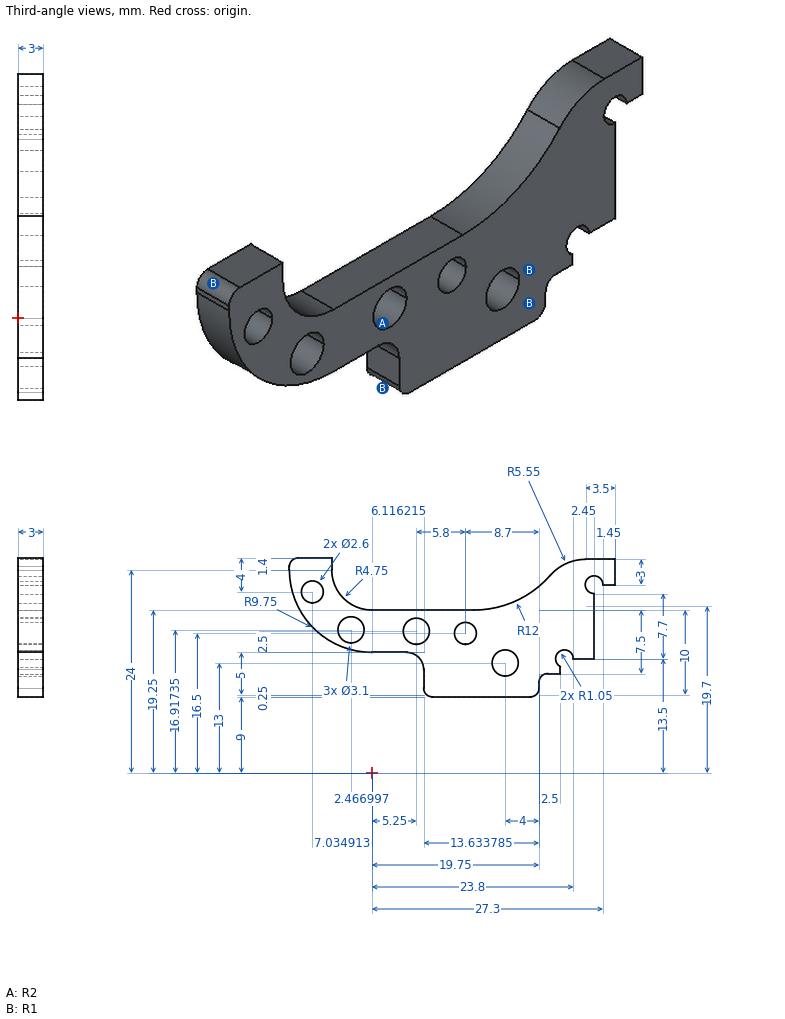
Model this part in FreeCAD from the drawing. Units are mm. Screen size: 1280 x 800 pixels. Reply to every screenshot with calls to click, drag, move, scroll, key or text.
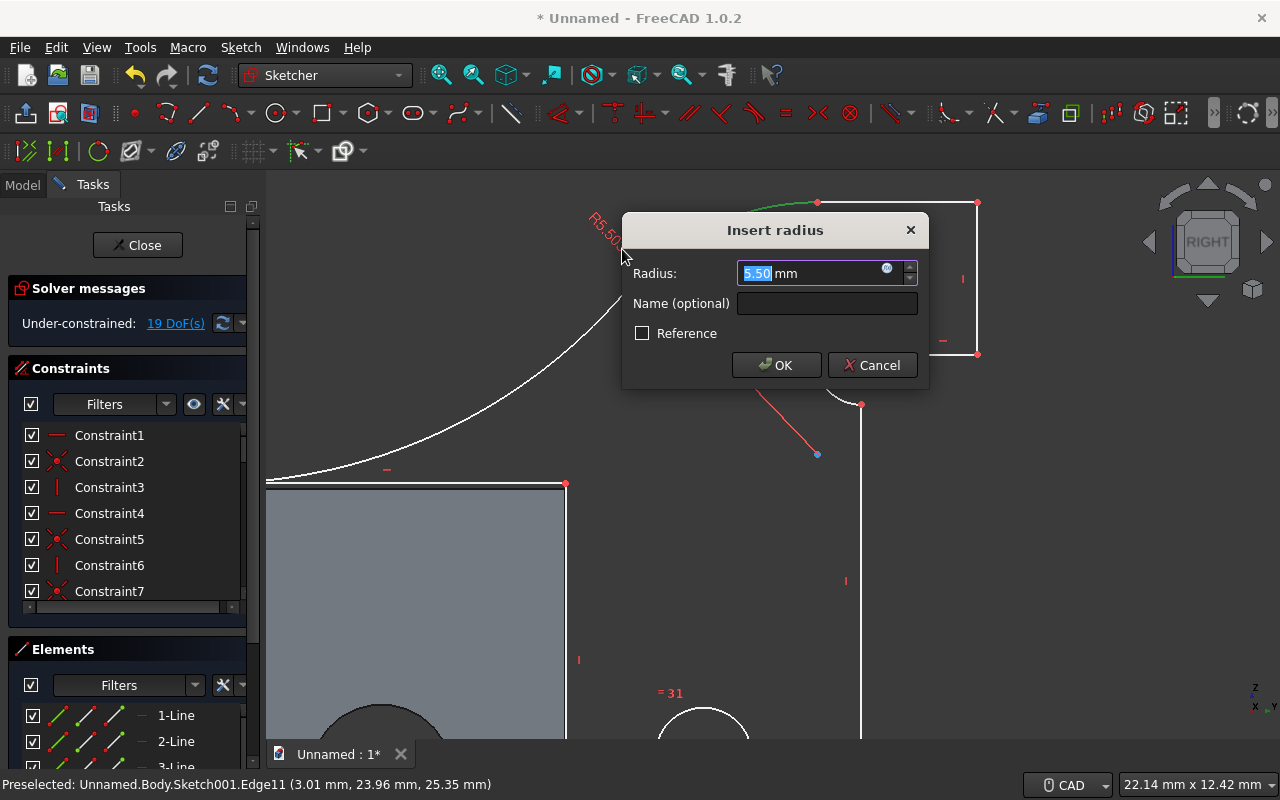
text(5.55)
key(Return)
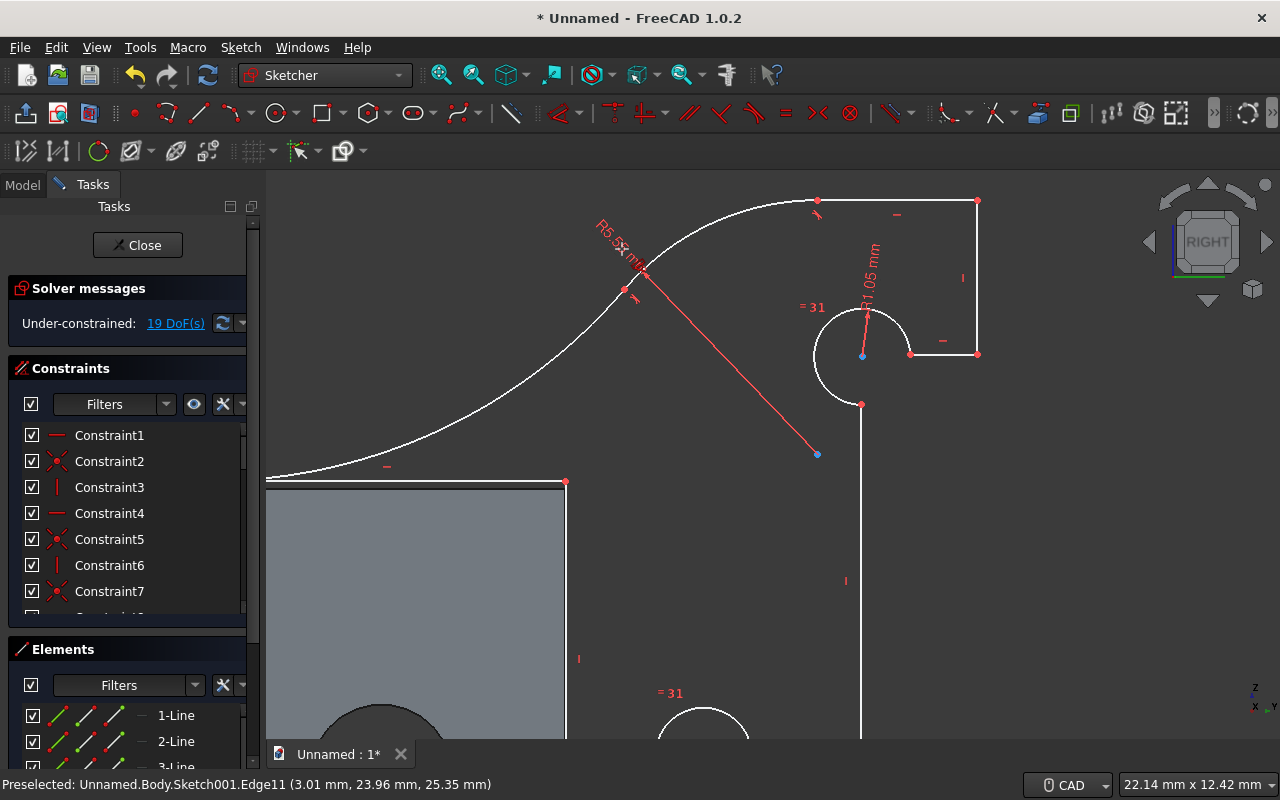
click(349, 463)
click(606, 355)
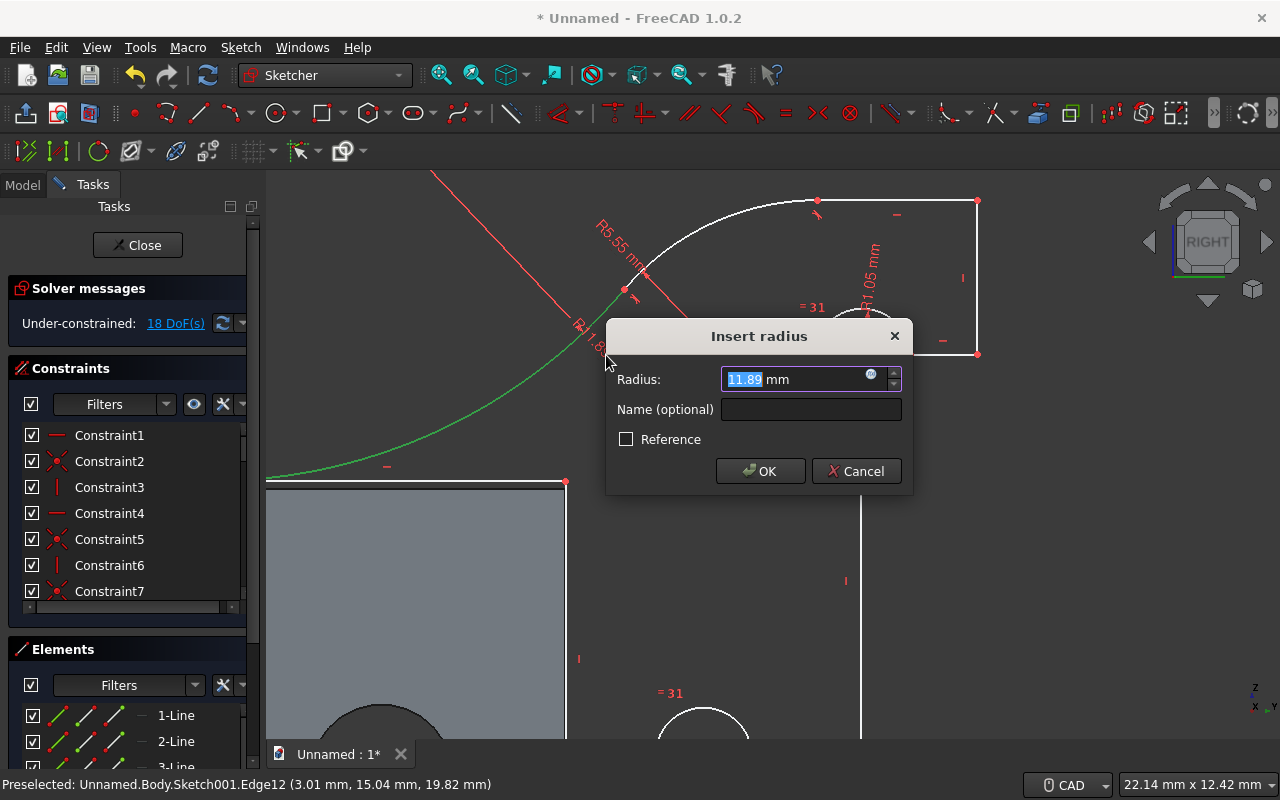
text(12)
key(Return)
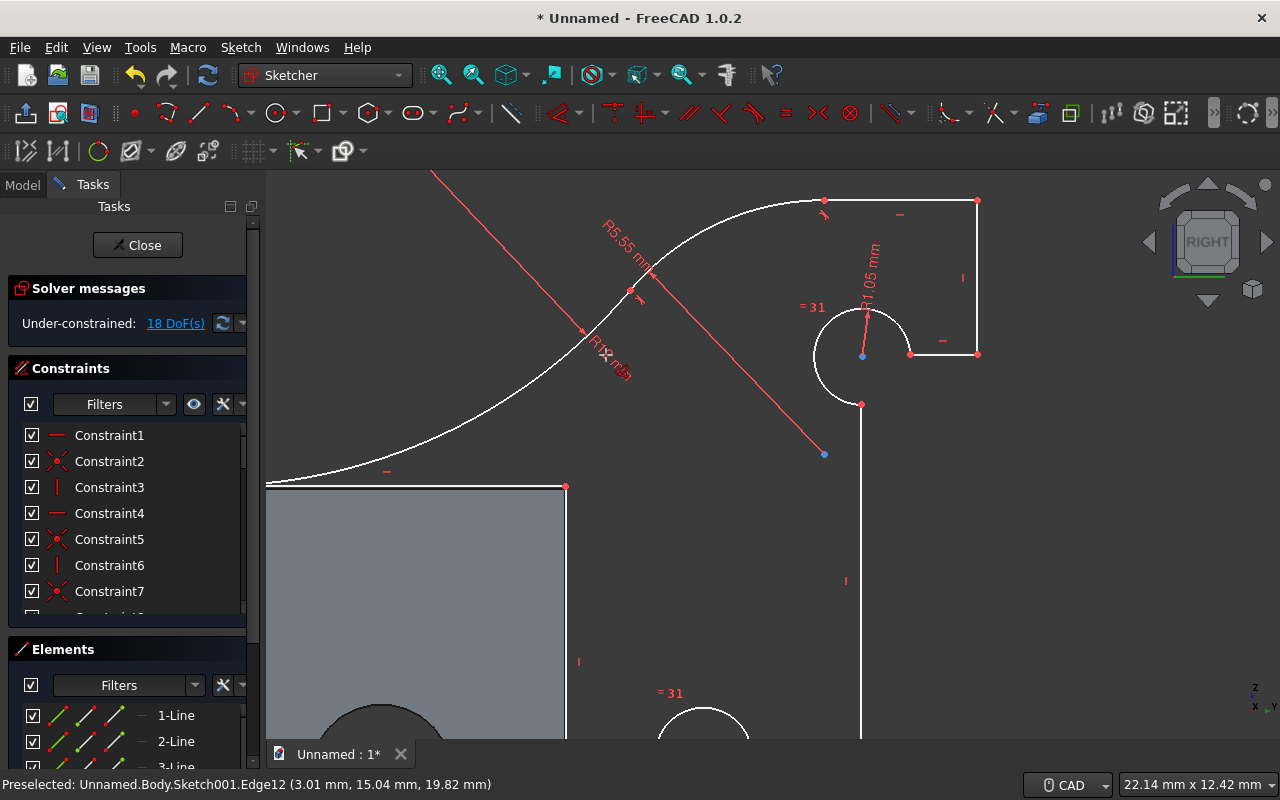
click(977, 308)
click(1011, 278)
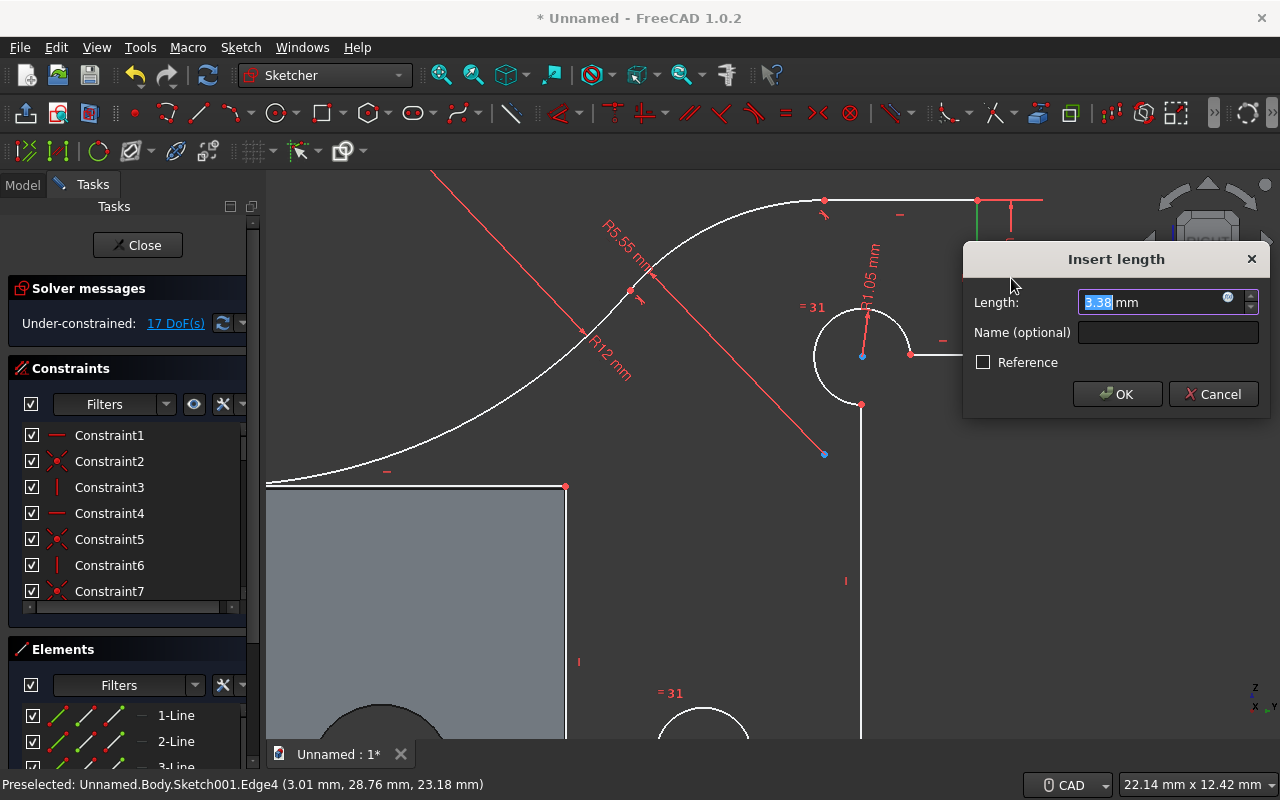
text(3)
key(Return)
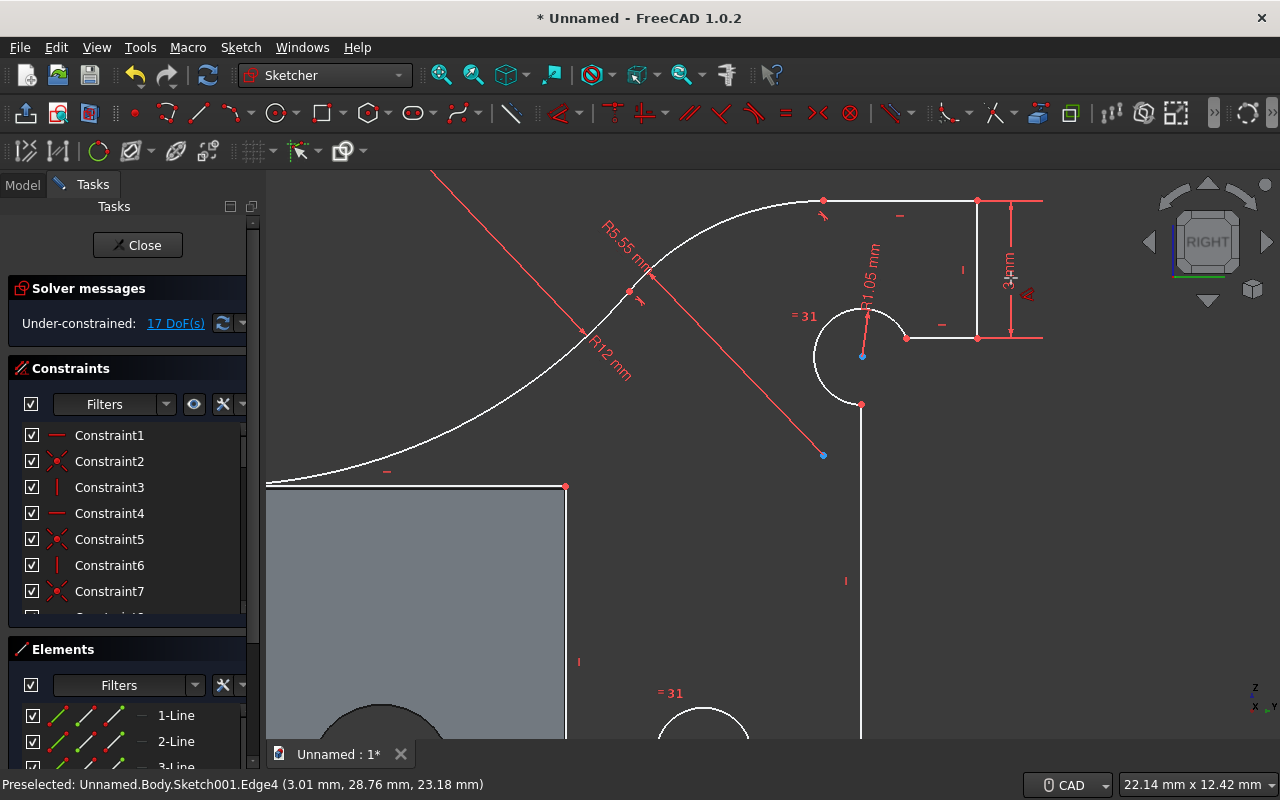
scroll(871, 309, down, 6)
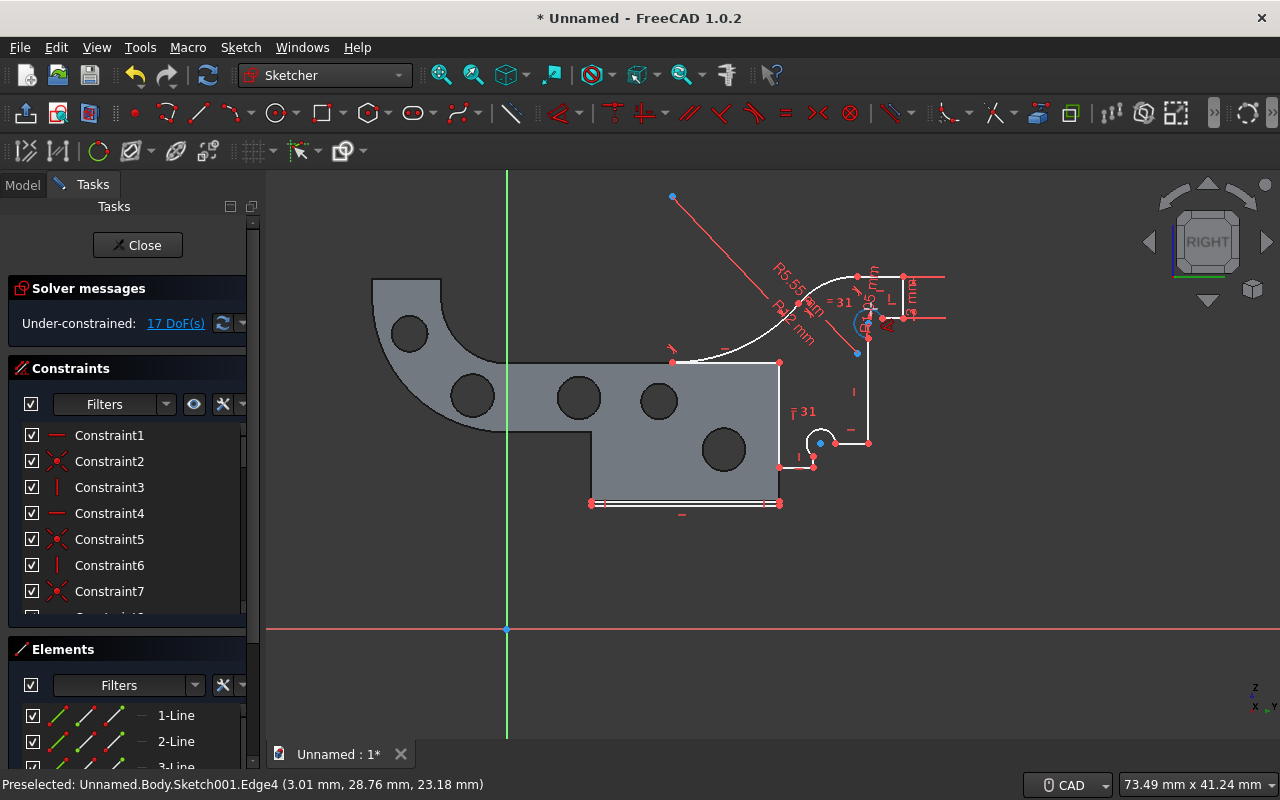
scroll(591, 506, up, 6)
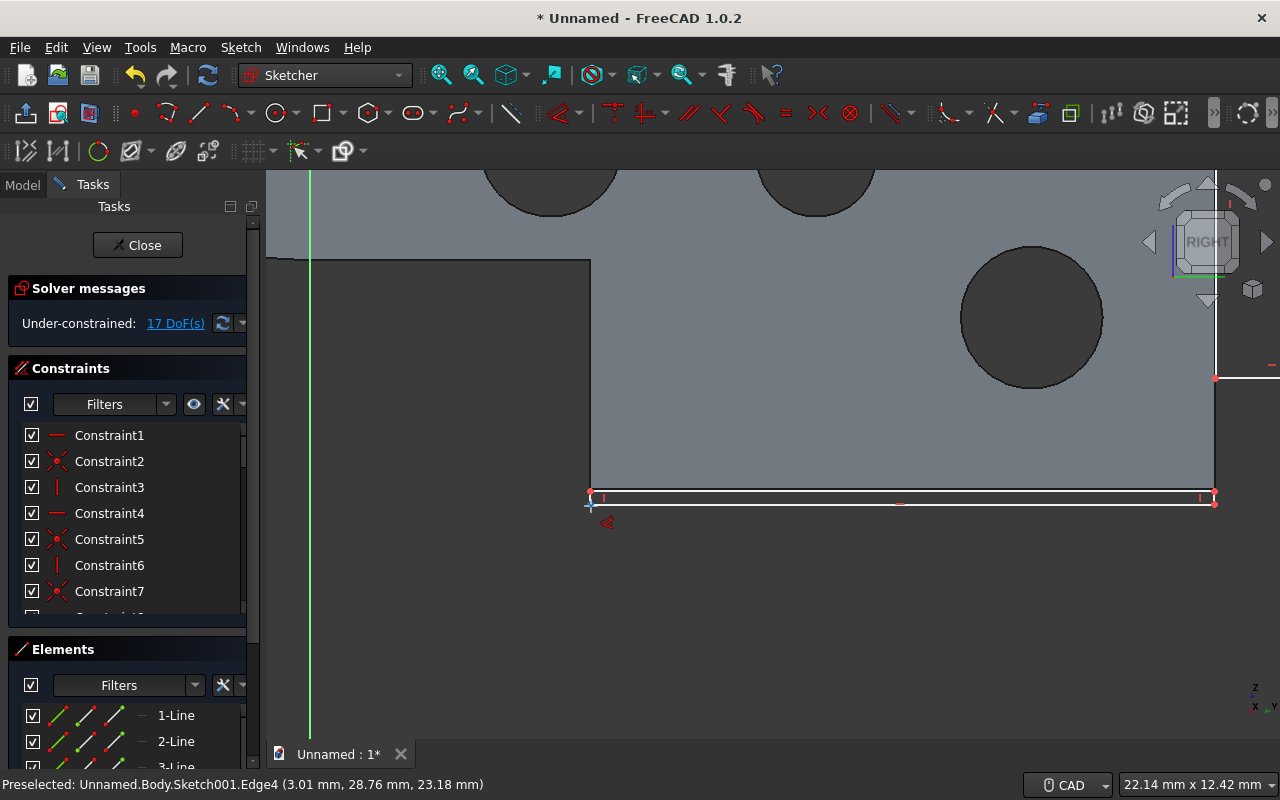
click(590, 505)
click(624, 608)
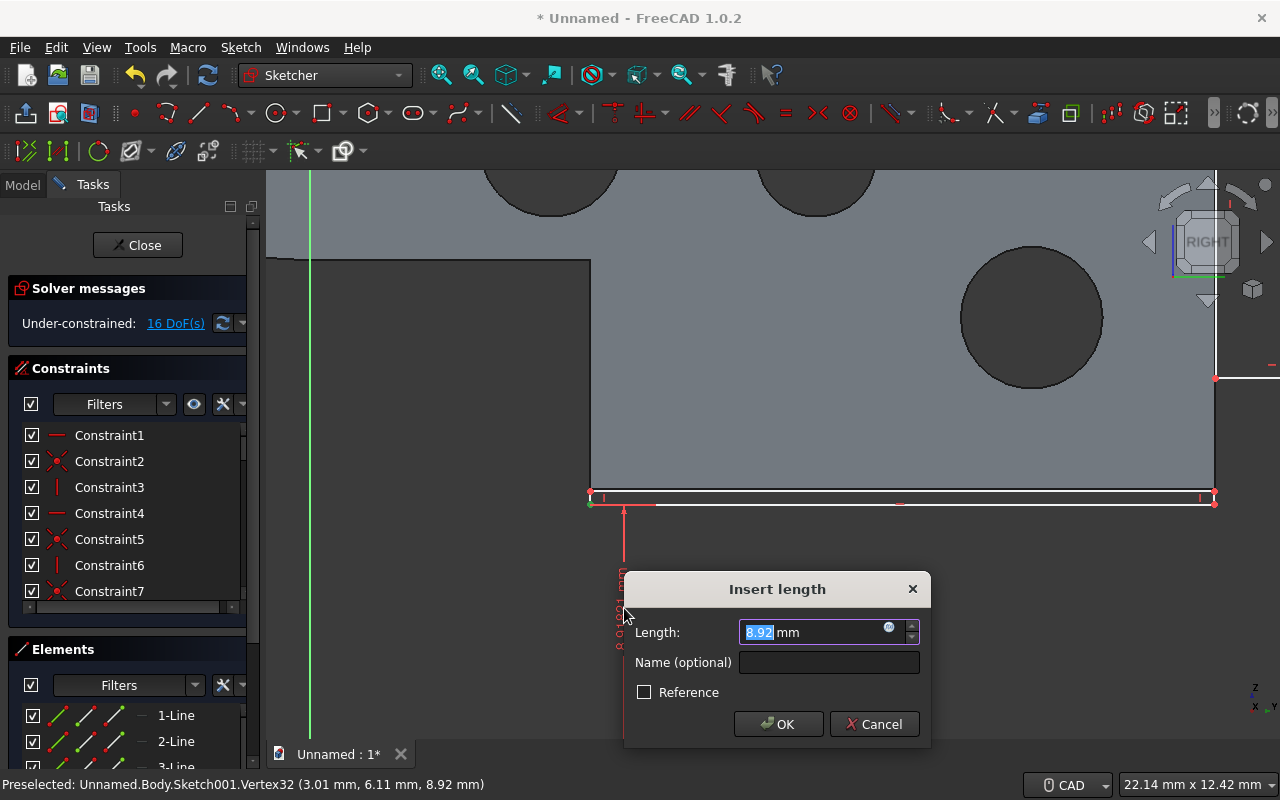
text(9)
key(Return)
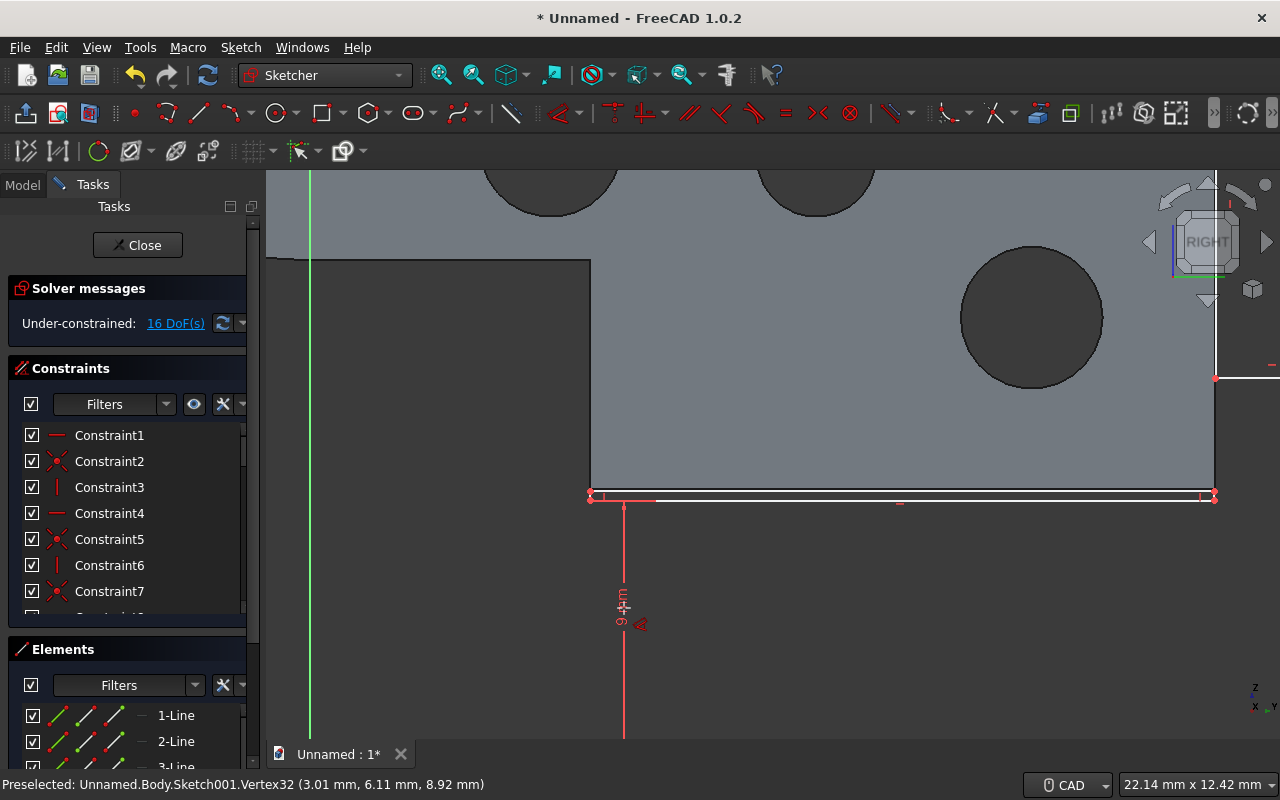
scroll(591, 506, down, 6)